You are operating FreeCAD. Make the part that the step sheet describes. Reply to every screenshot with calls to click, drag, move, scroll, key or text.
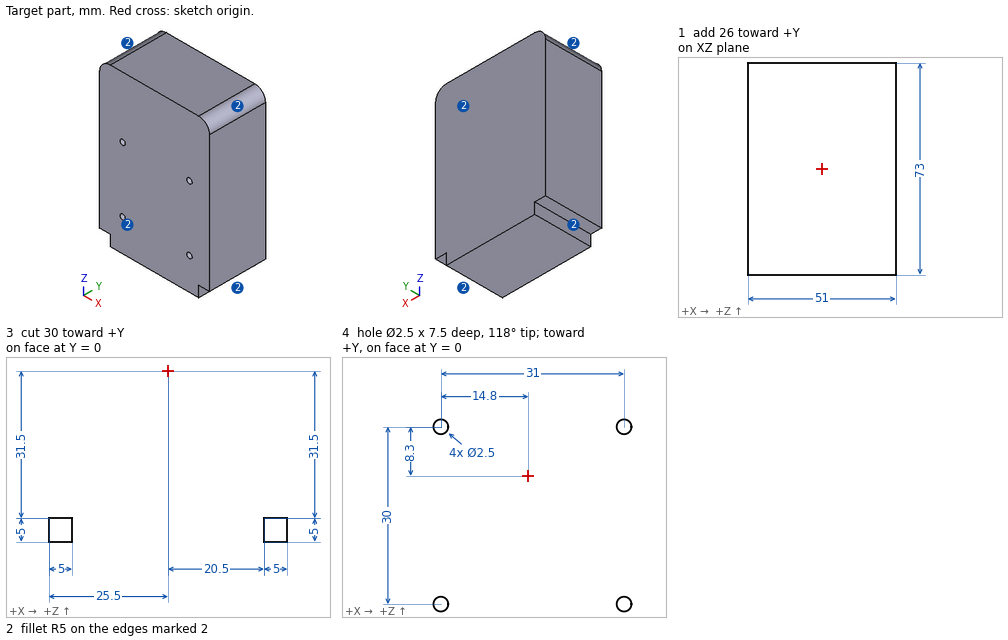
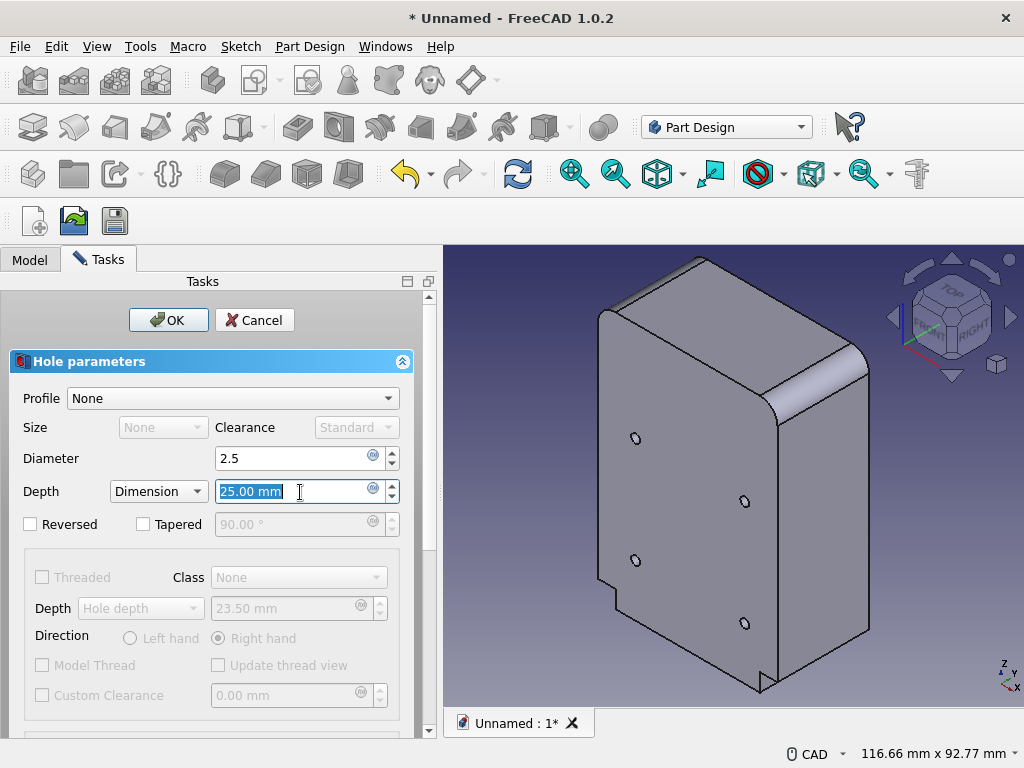
text(7.5)
key(Tab)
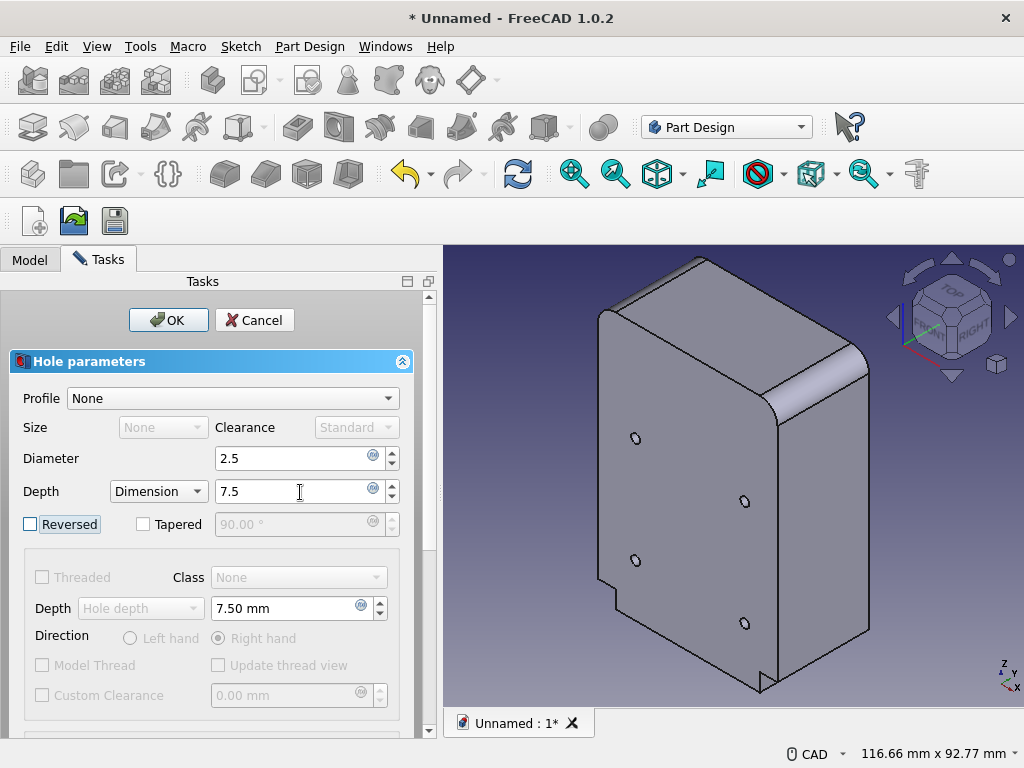
click(169, 320)